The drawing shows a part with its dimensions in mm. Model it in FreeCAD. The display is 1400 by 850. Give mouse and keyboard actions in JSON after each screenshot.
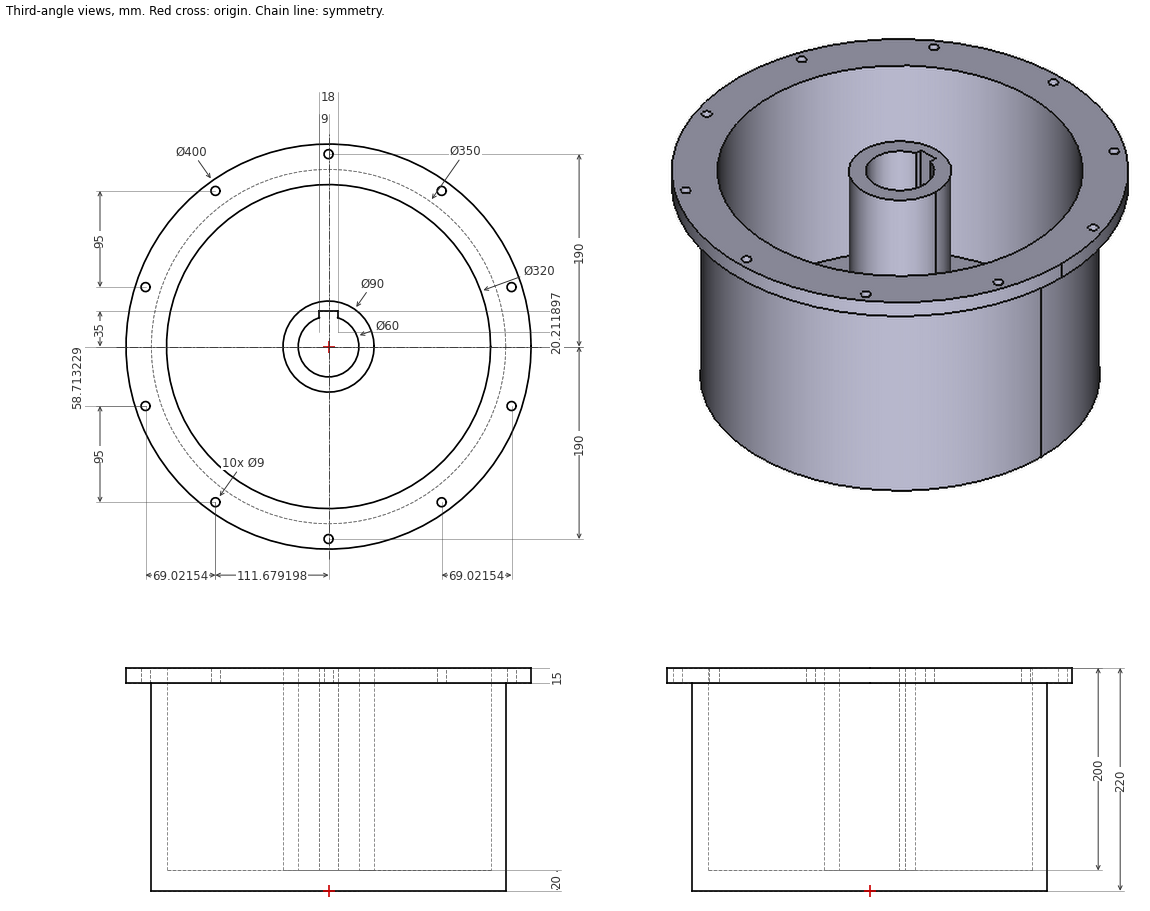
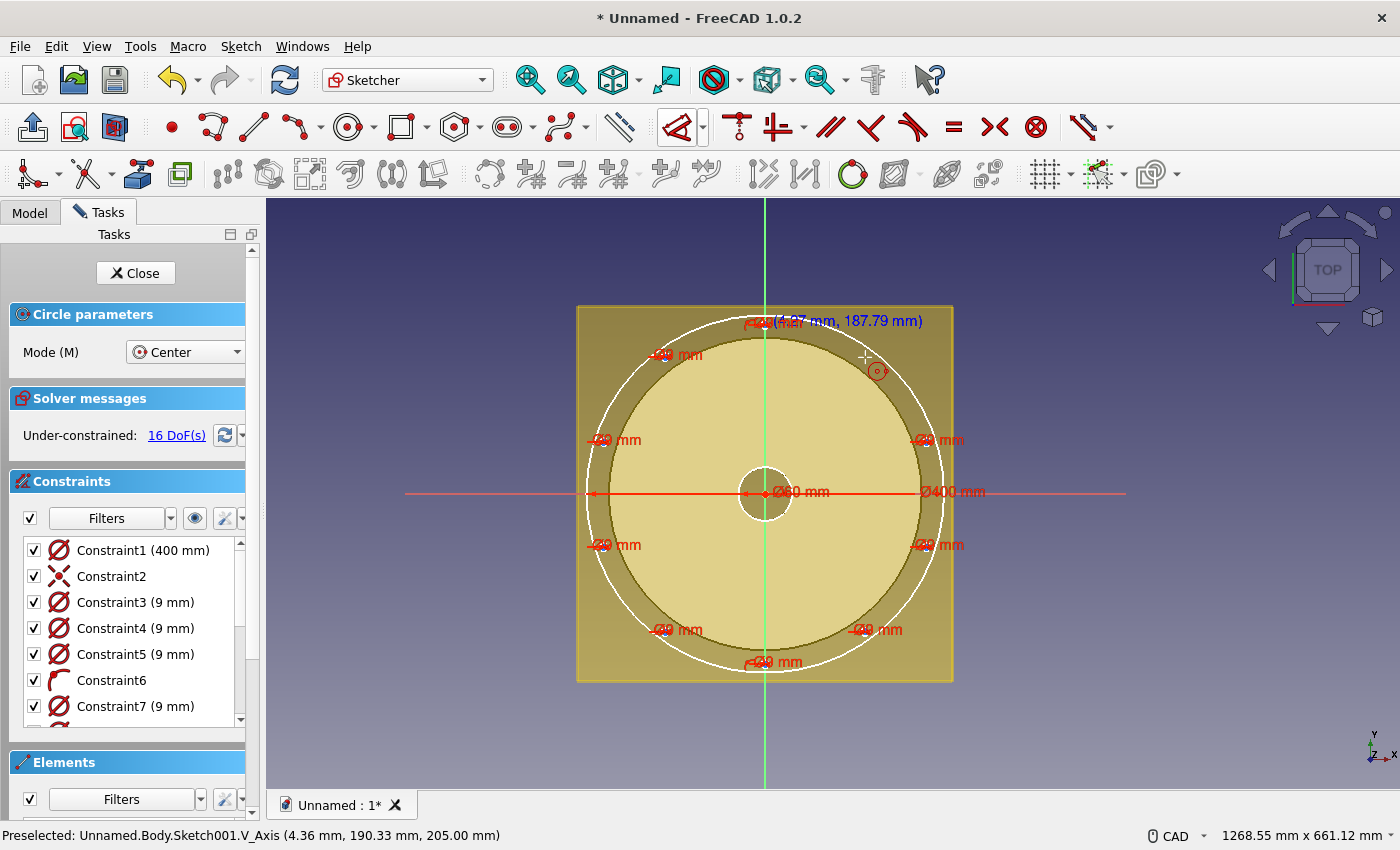
{"action": "scroll", "coordinate": [865, 357], "scroll_direction": "up", "scroll_amount": 3}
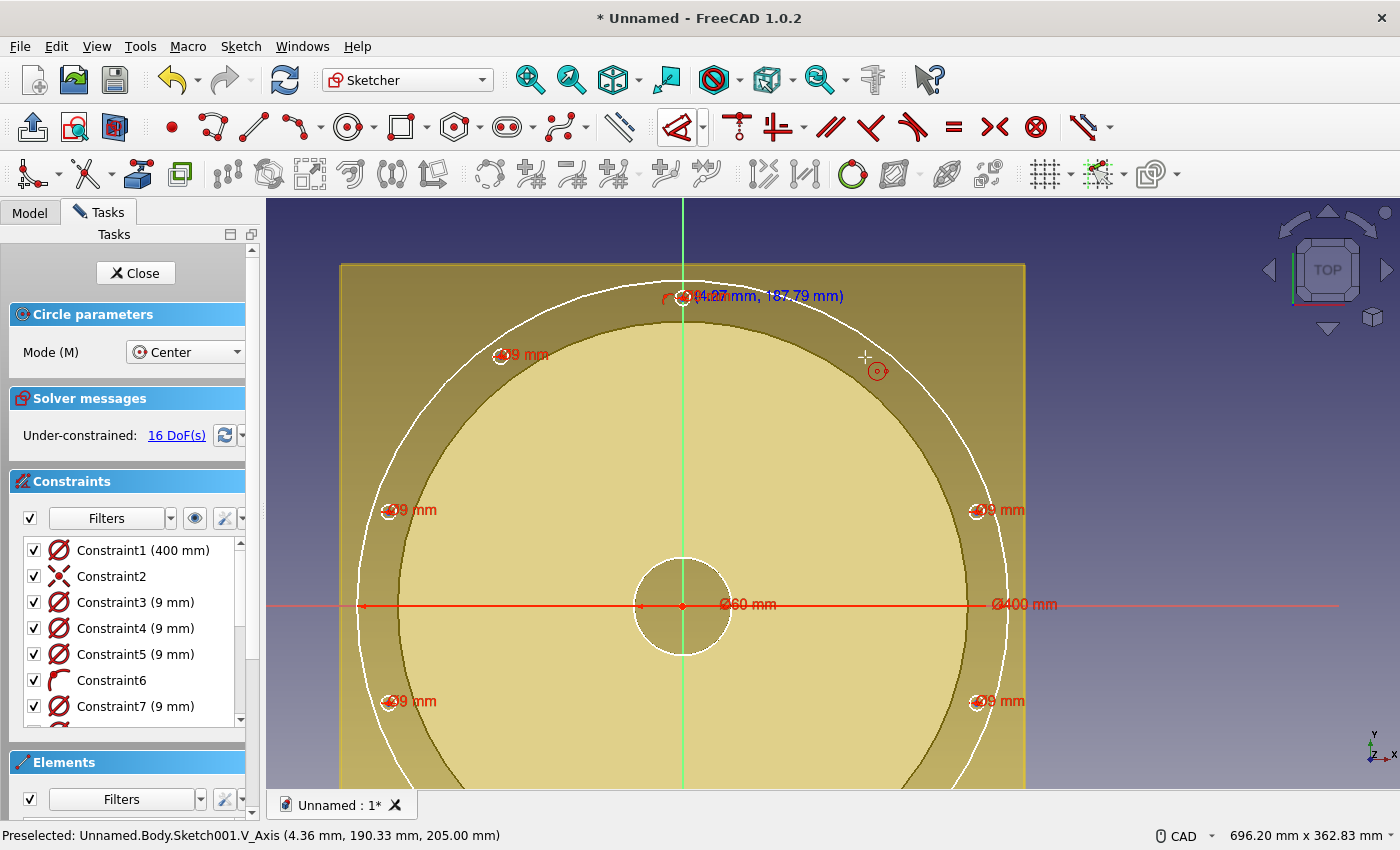
{"action": "left_click", "coordinate": [865, 356]}
{"action": "mouse_move", "coordinate": [860, 351]}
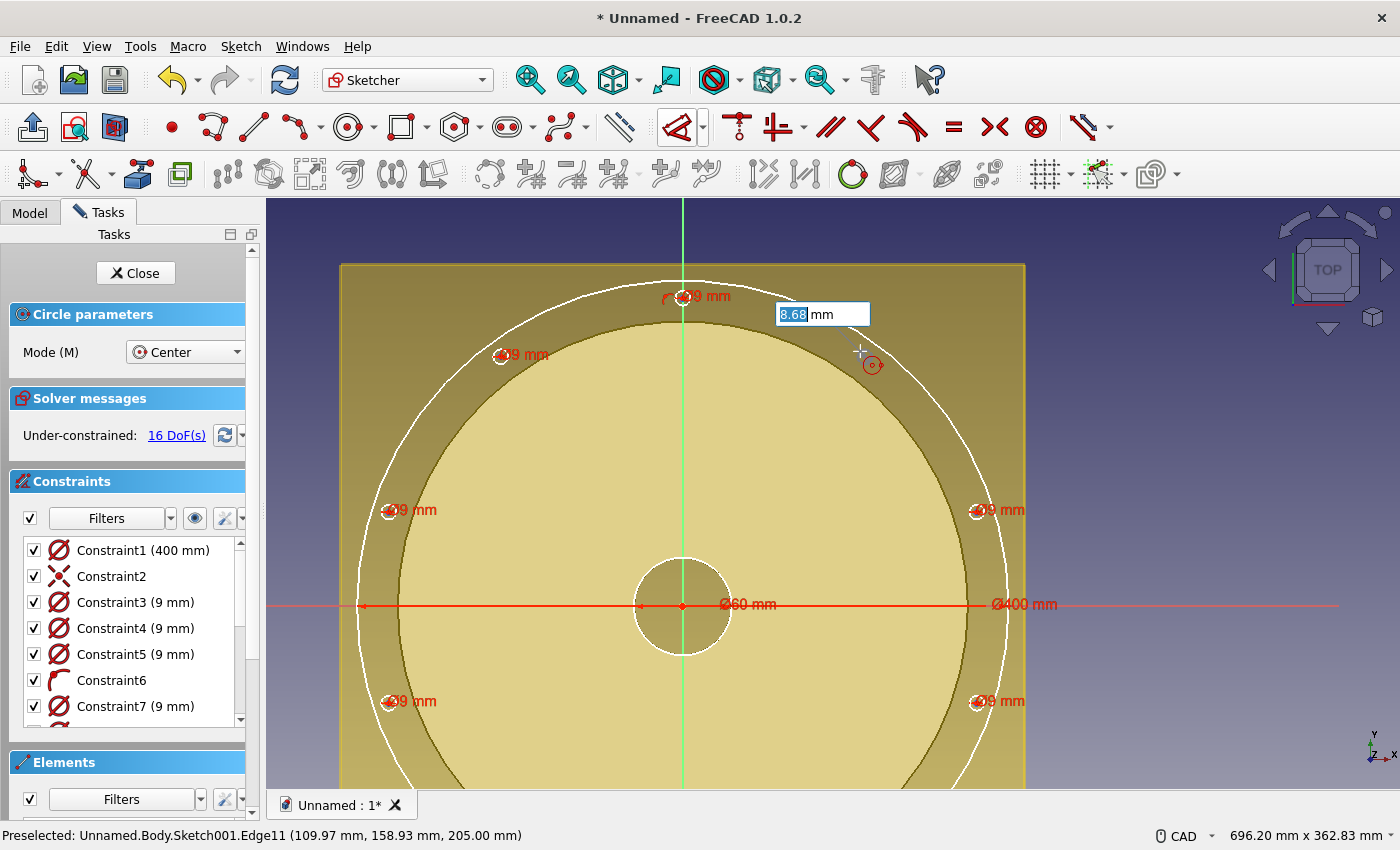
{"action": "type", "text": "9"}
{"action": "key", "text": "Return"}
{"action": "key", "text": "Escape"}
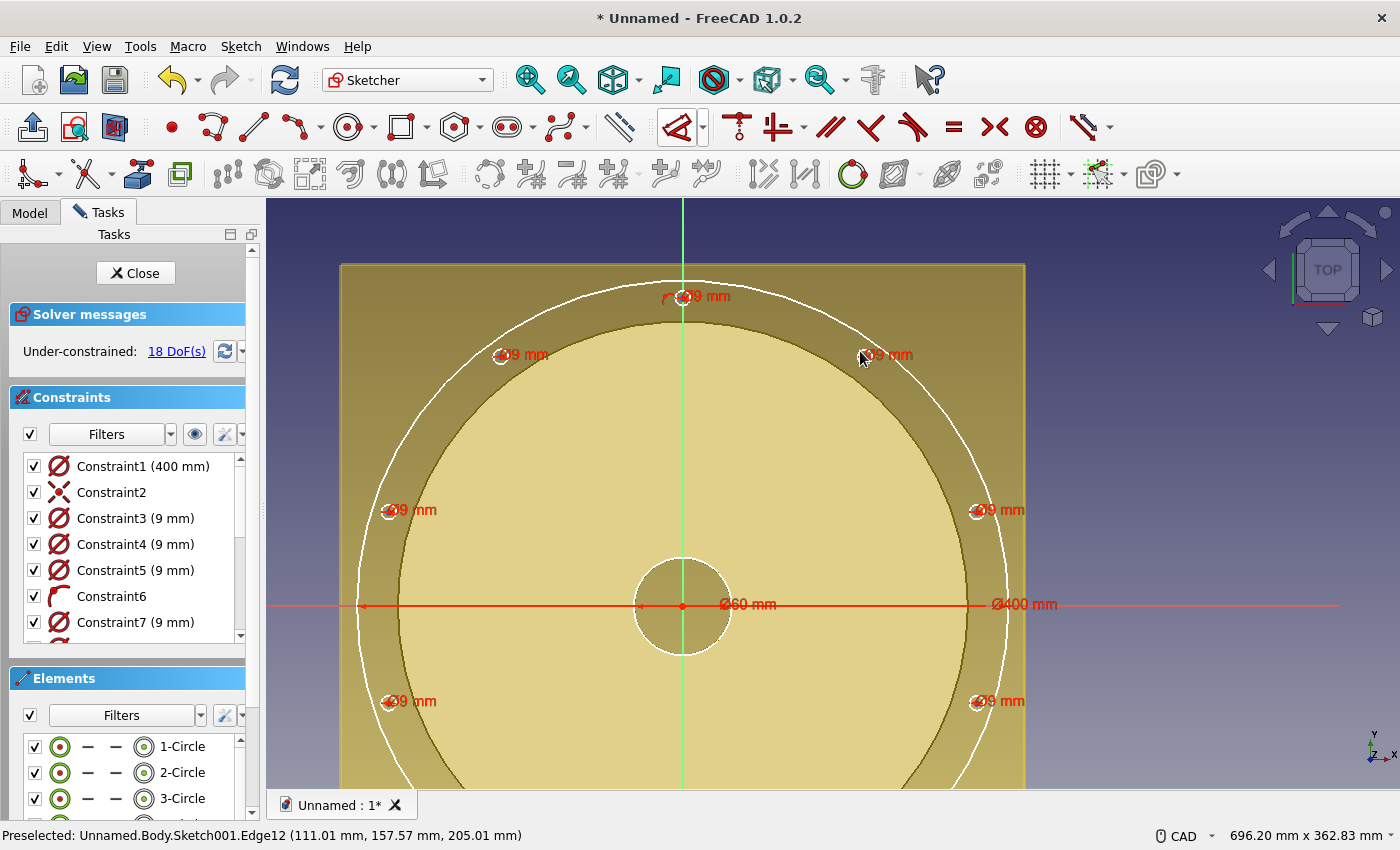
{"action": "scroll", "coordinate": [864, 356], "scroll_direction": "down", "scroll_amount": 3}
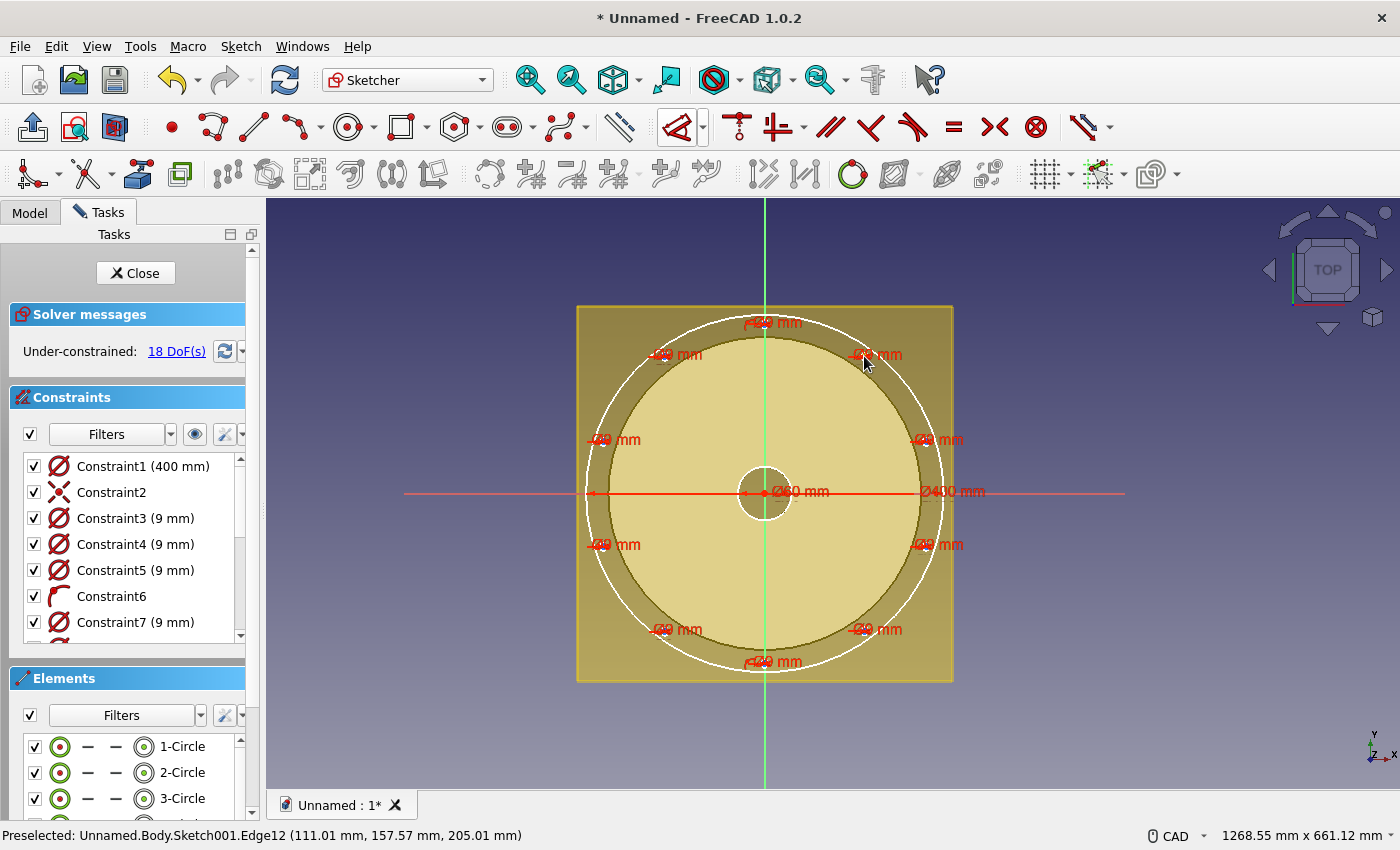
{"action": "left_click", "coordinate": [665, 632]}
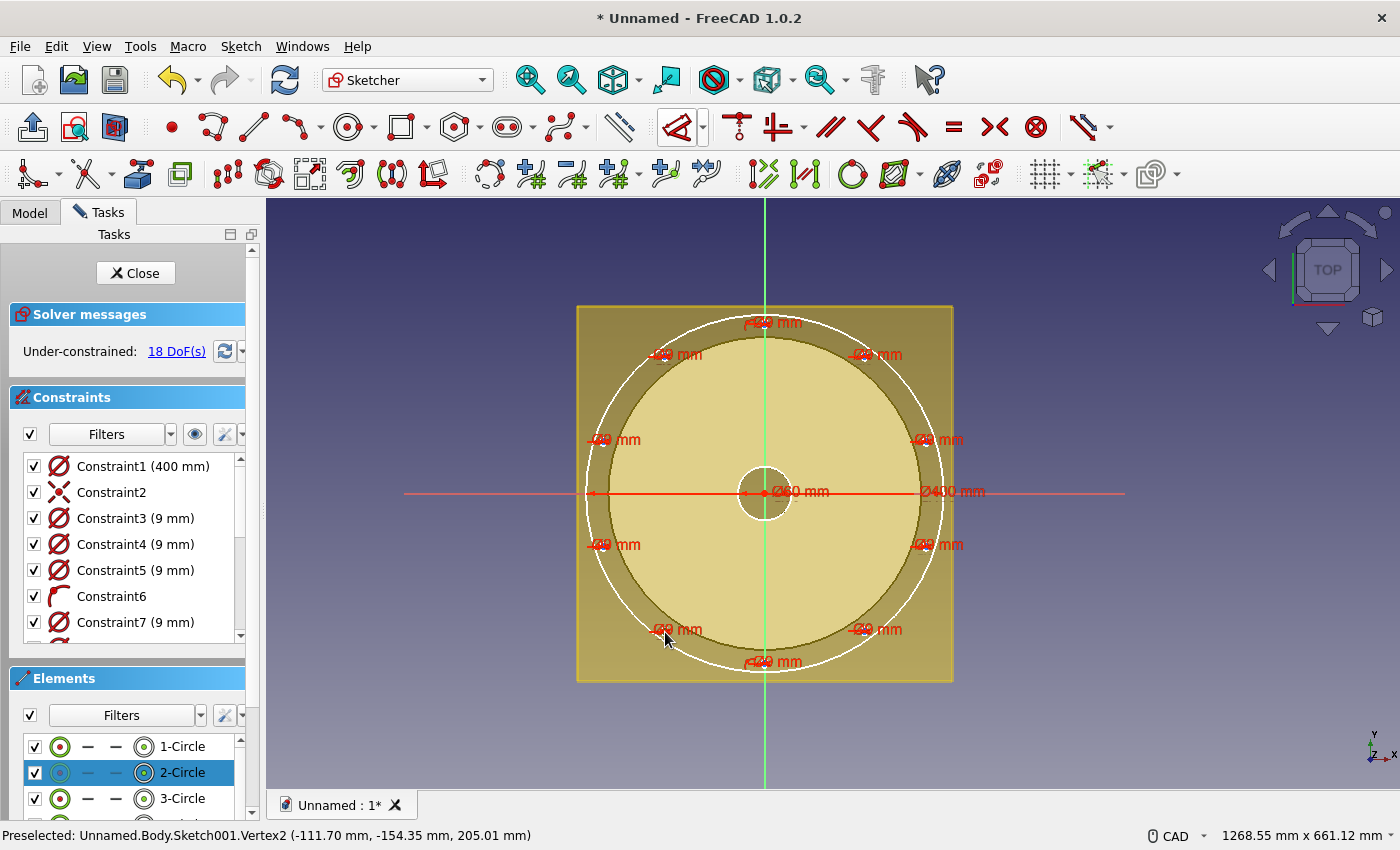
{"action": "left_click", "coordinate": [865, 631]}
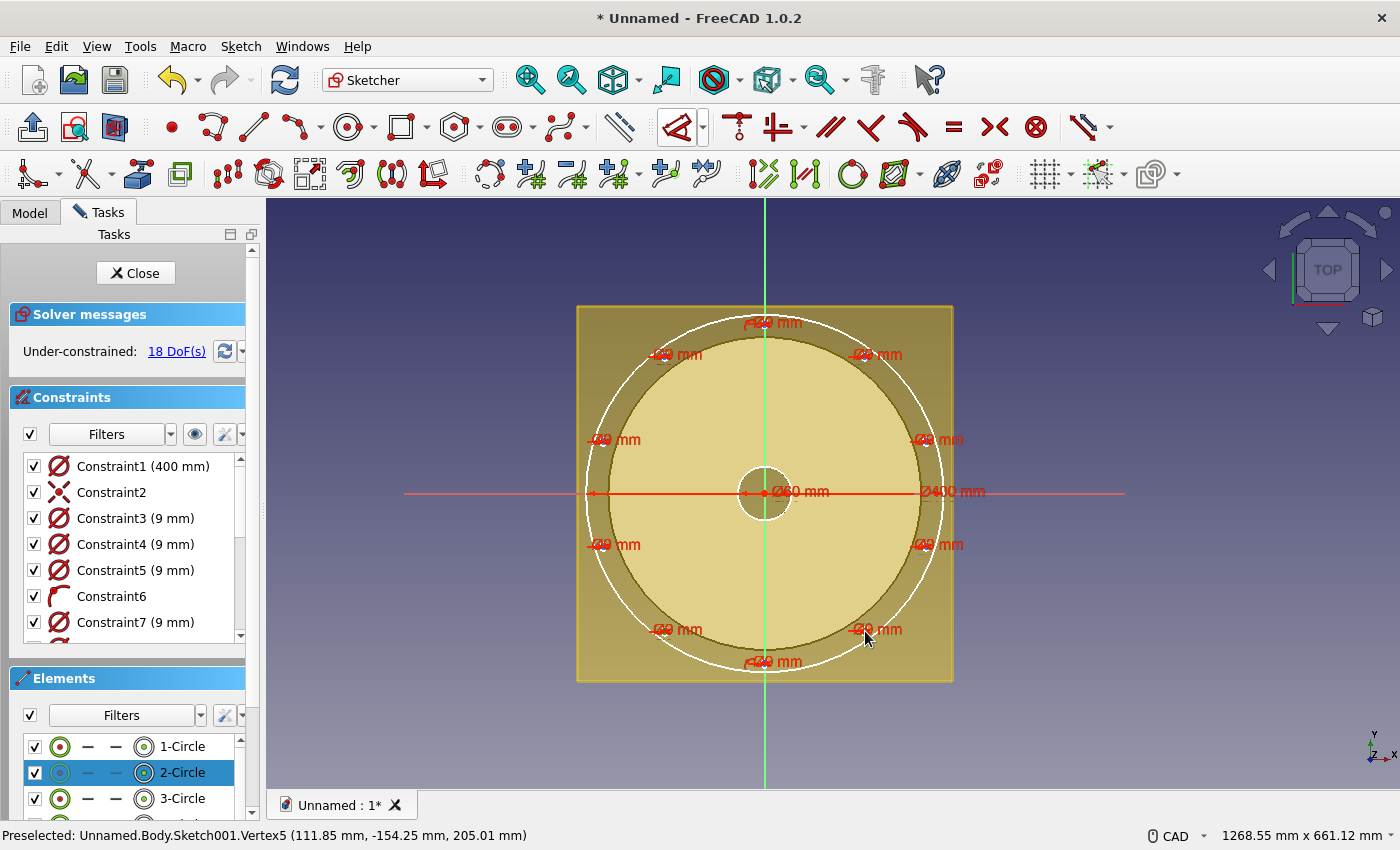
{"action": "left_click", "coordinate": [804, 128]}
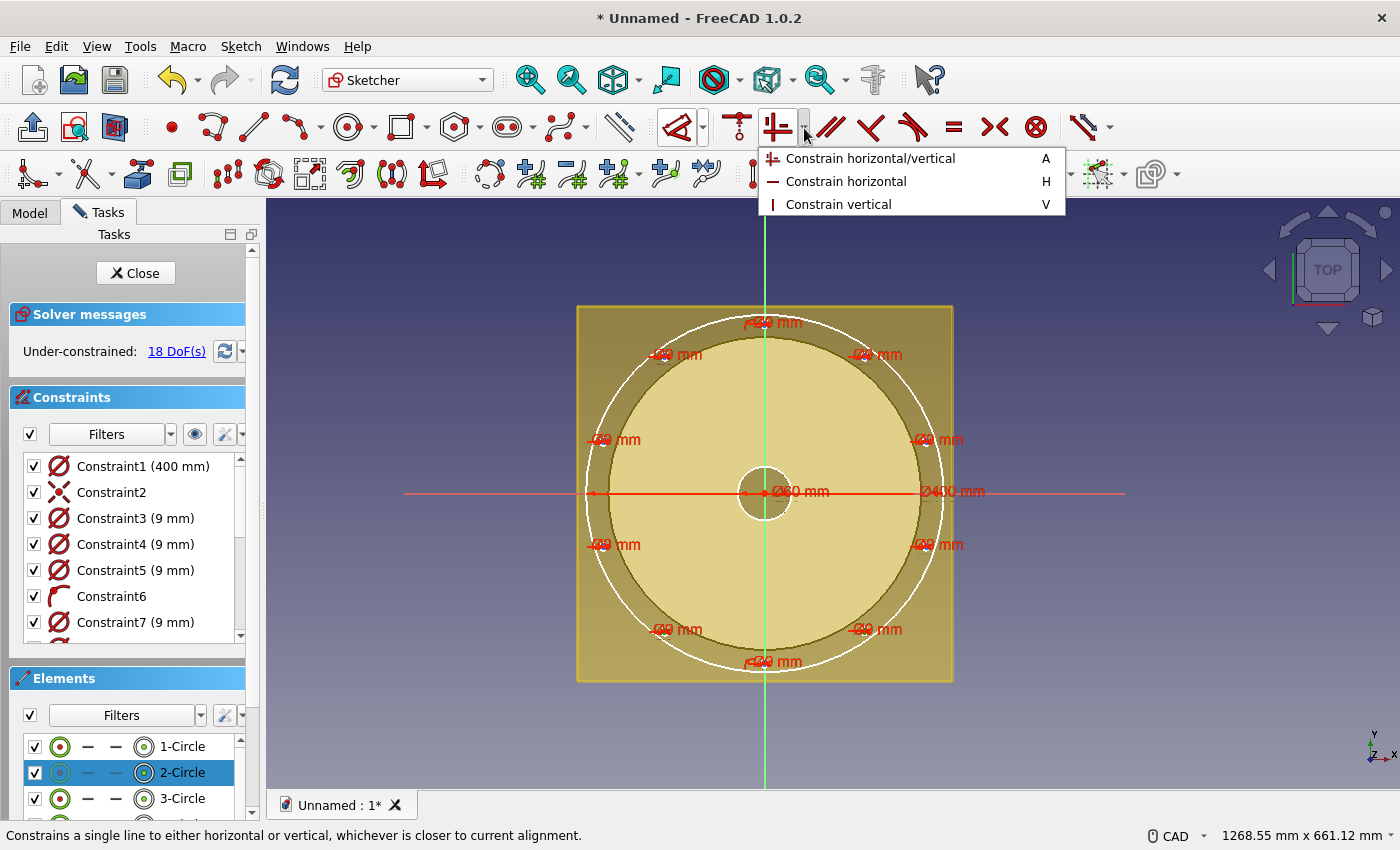
{"action": "left_click", "coordinate": [912, 182]}